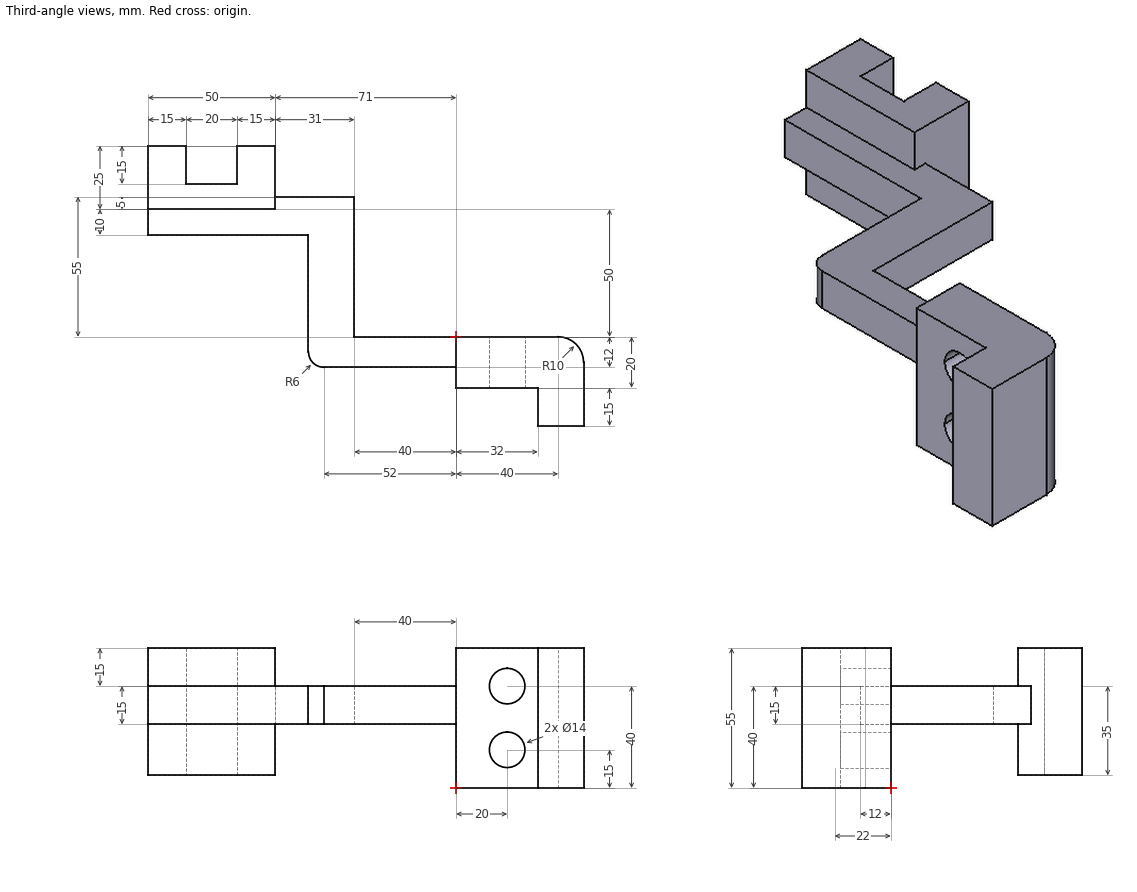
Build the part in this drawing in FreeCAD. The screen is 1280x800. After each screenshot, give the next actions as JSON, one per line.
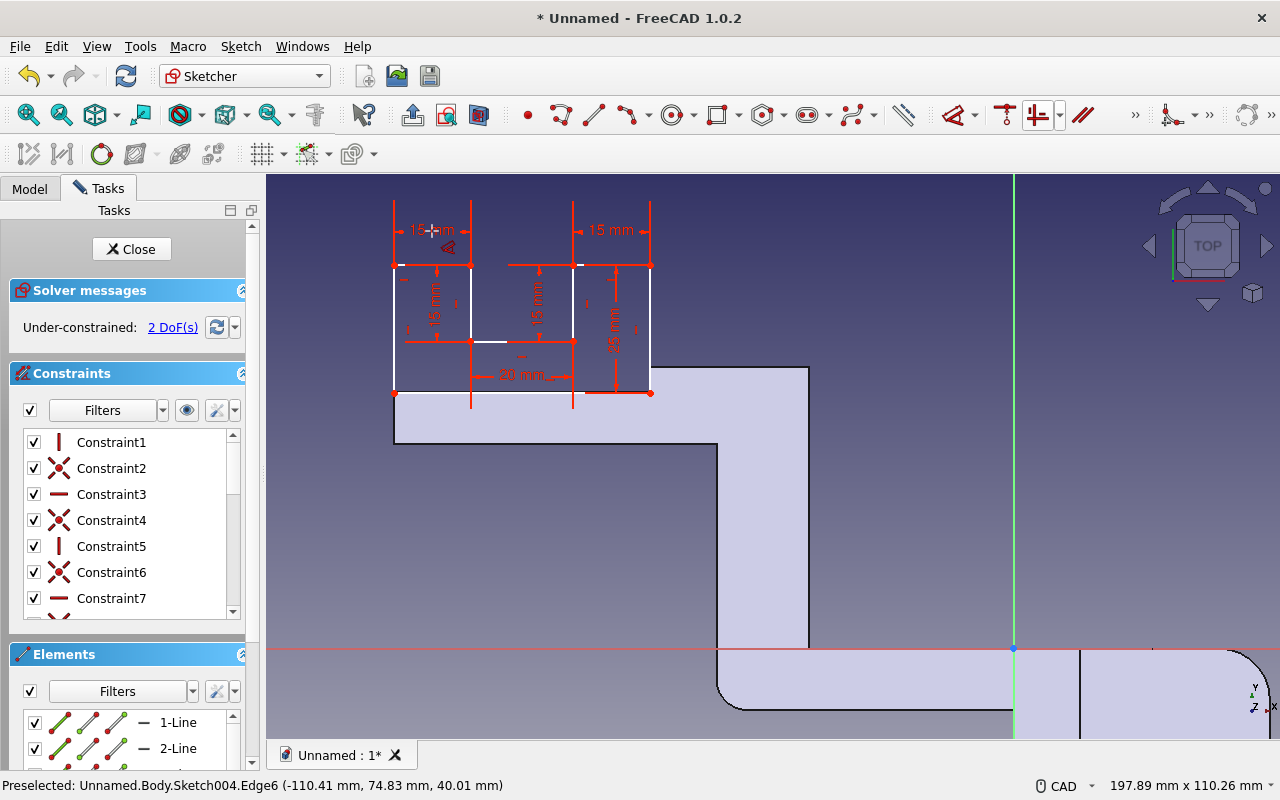
{"action": "left_click", "coordinate": [650, 393]}
{"action": "left_click", "coordinate": [832, 683]}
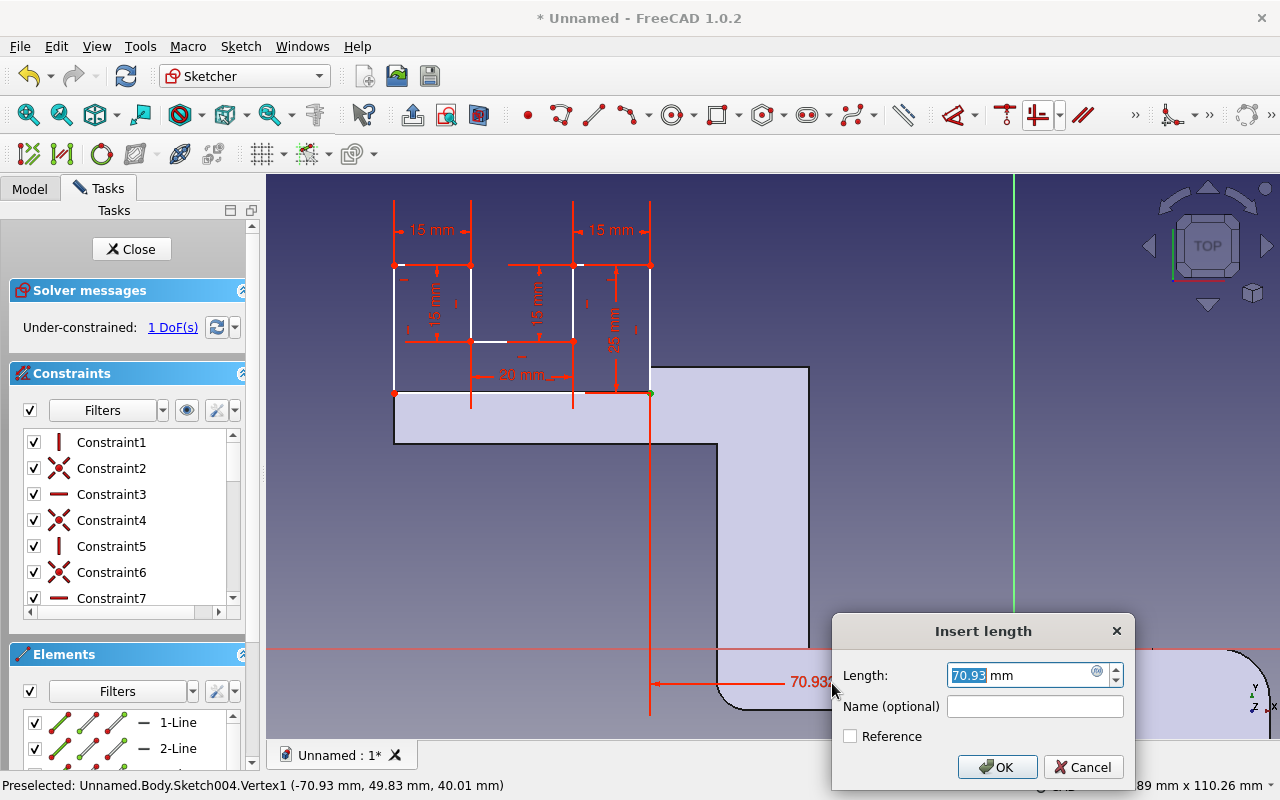
{"action": "type", "text": "71"}
{"action": "key", "text": "Return"}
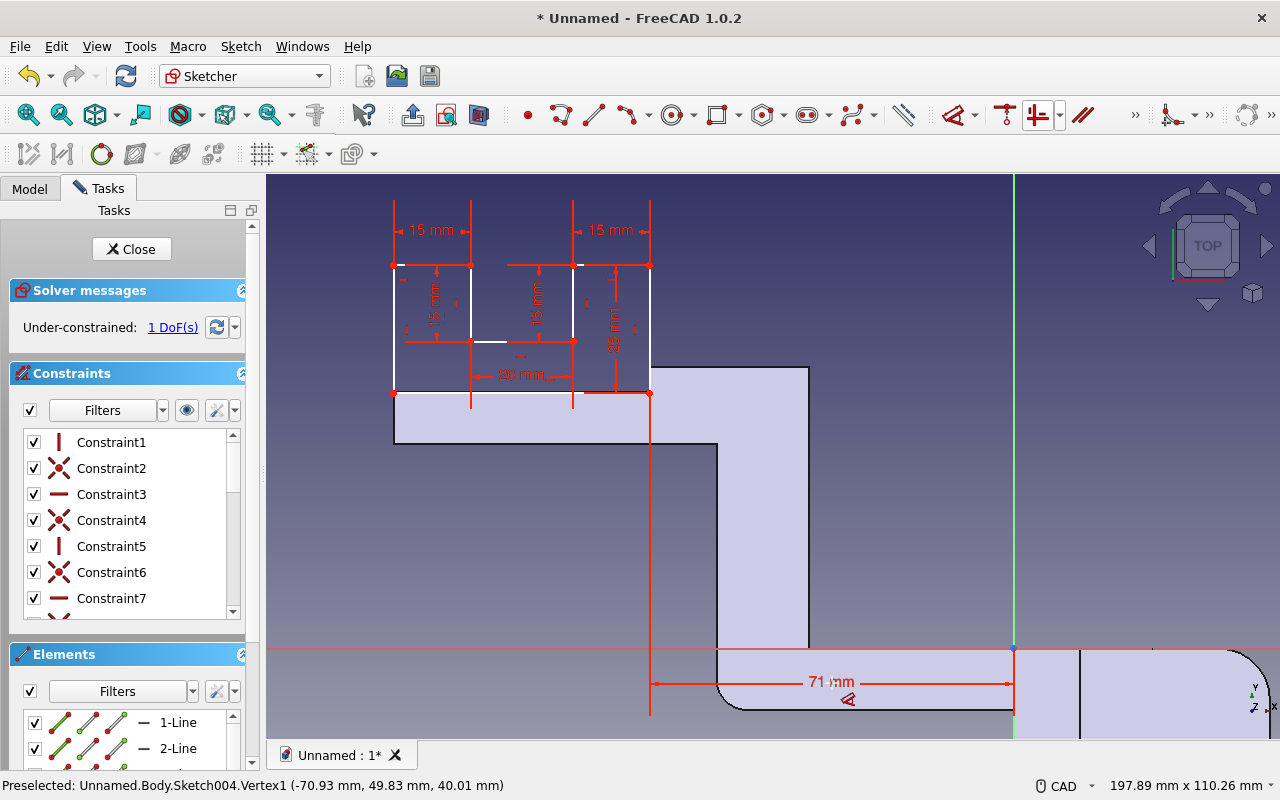
{"action": "left_click", "coordinate": [650, 393]}
{"action": "left_click", "coordinate": [1048, 521]}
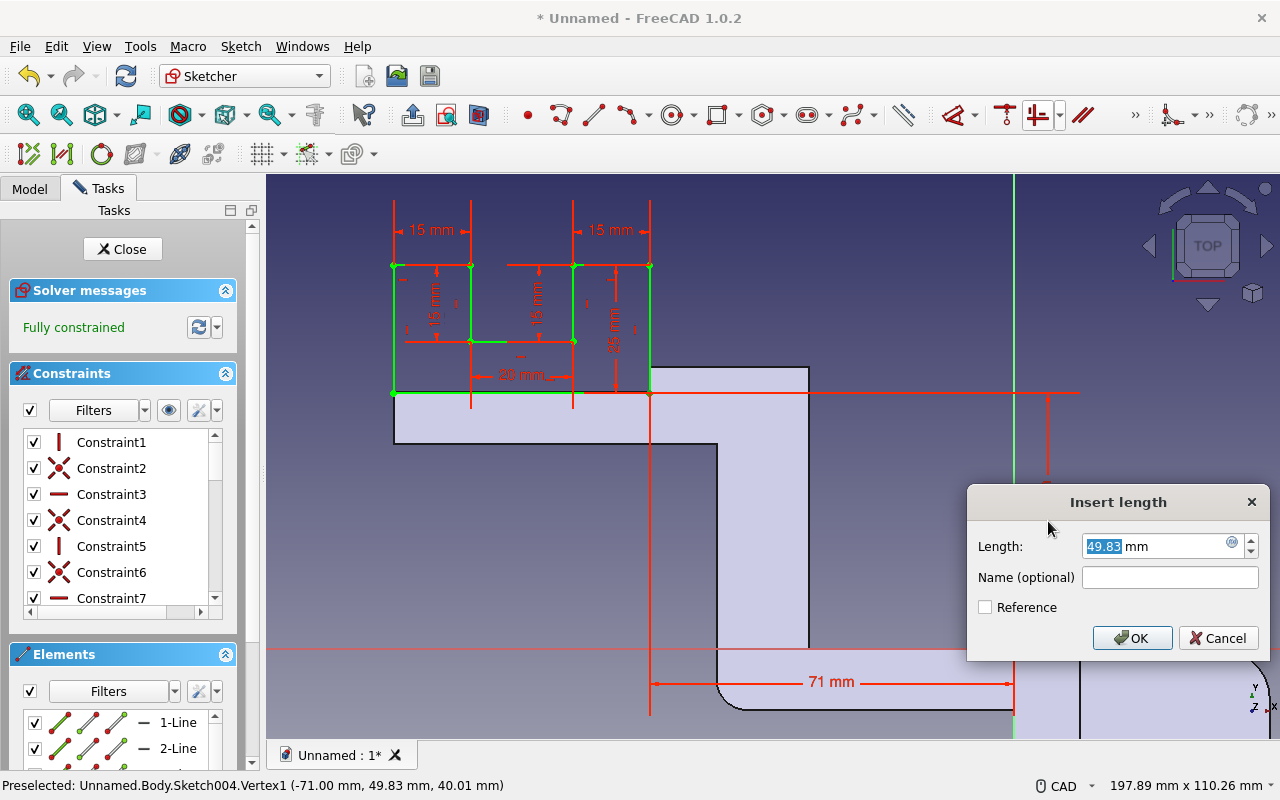
{"action": "type", "text": "50"}
{"action": "key", "text": "Return"}
{"action": "key", "text": "Escape"}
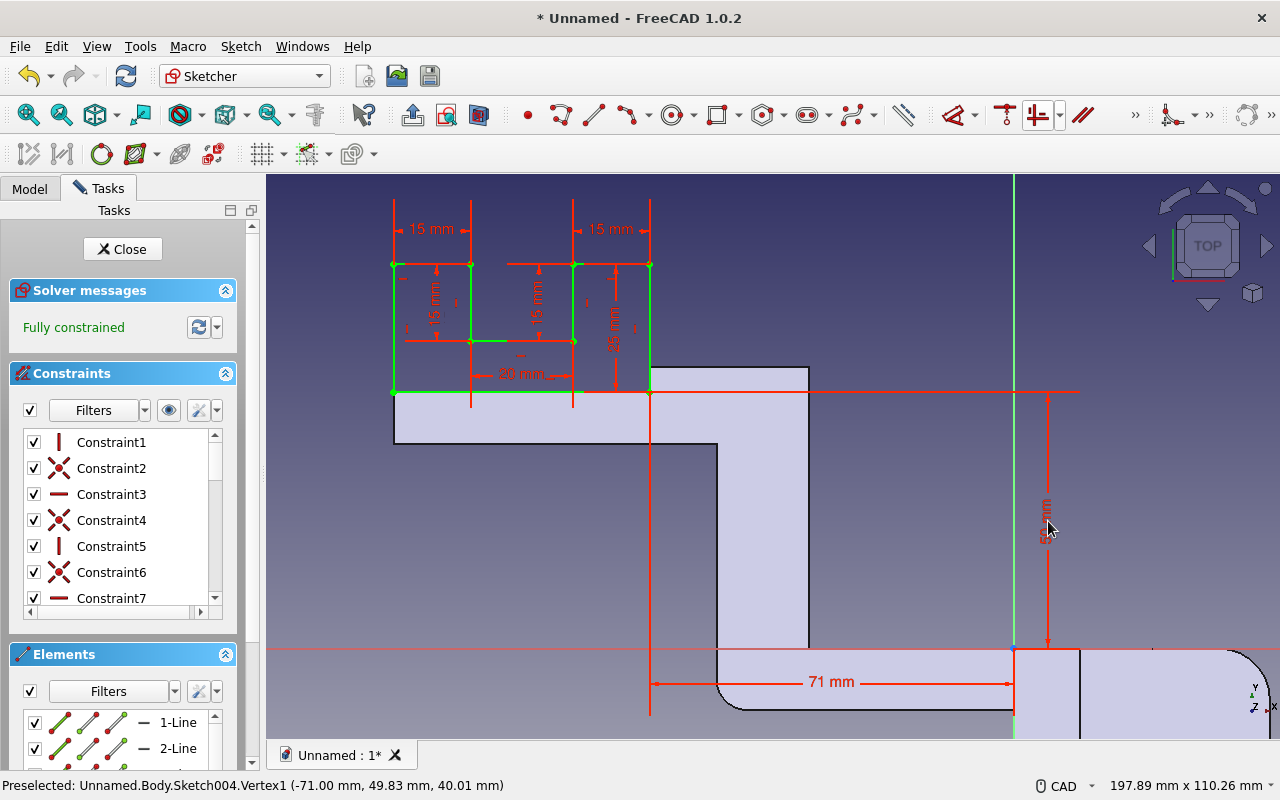
{"action": "left_click", "coordinate": [123, 249]}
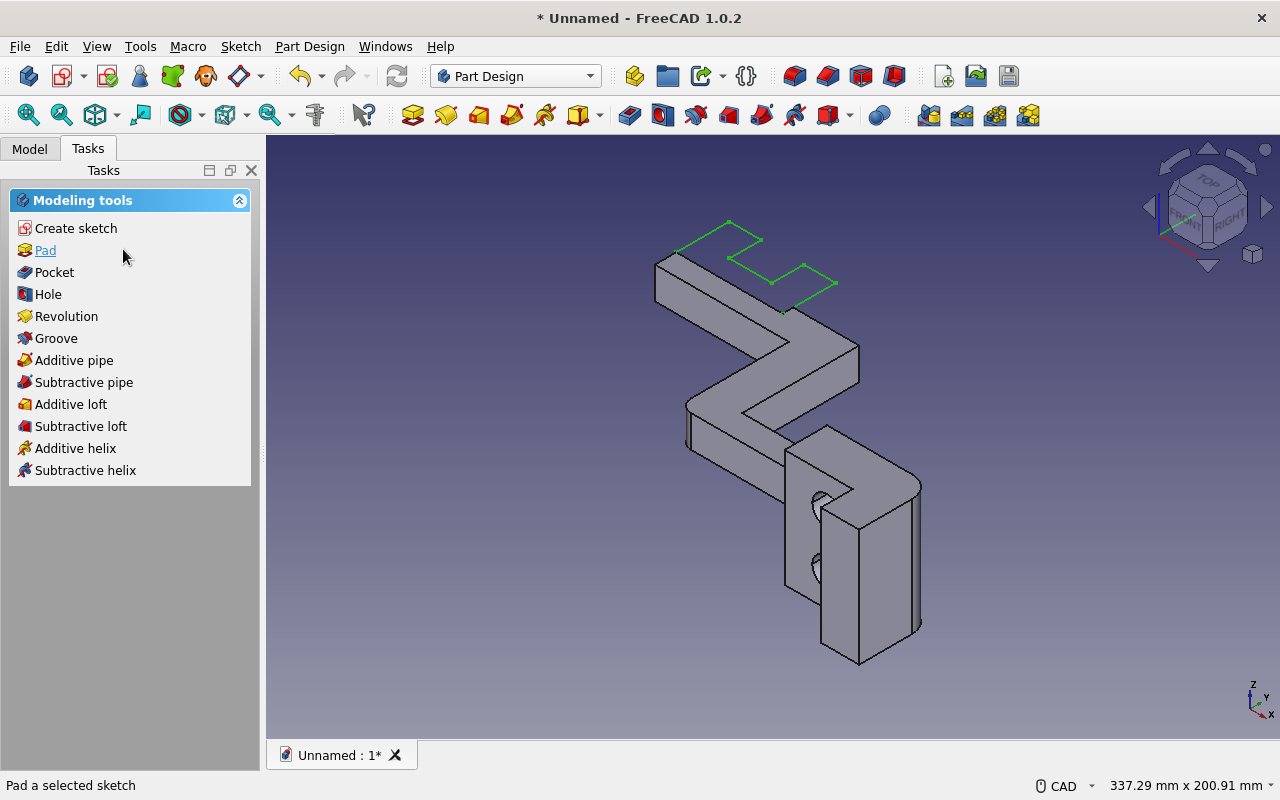
{"action": "left_click", "coordinate": [413, 116]}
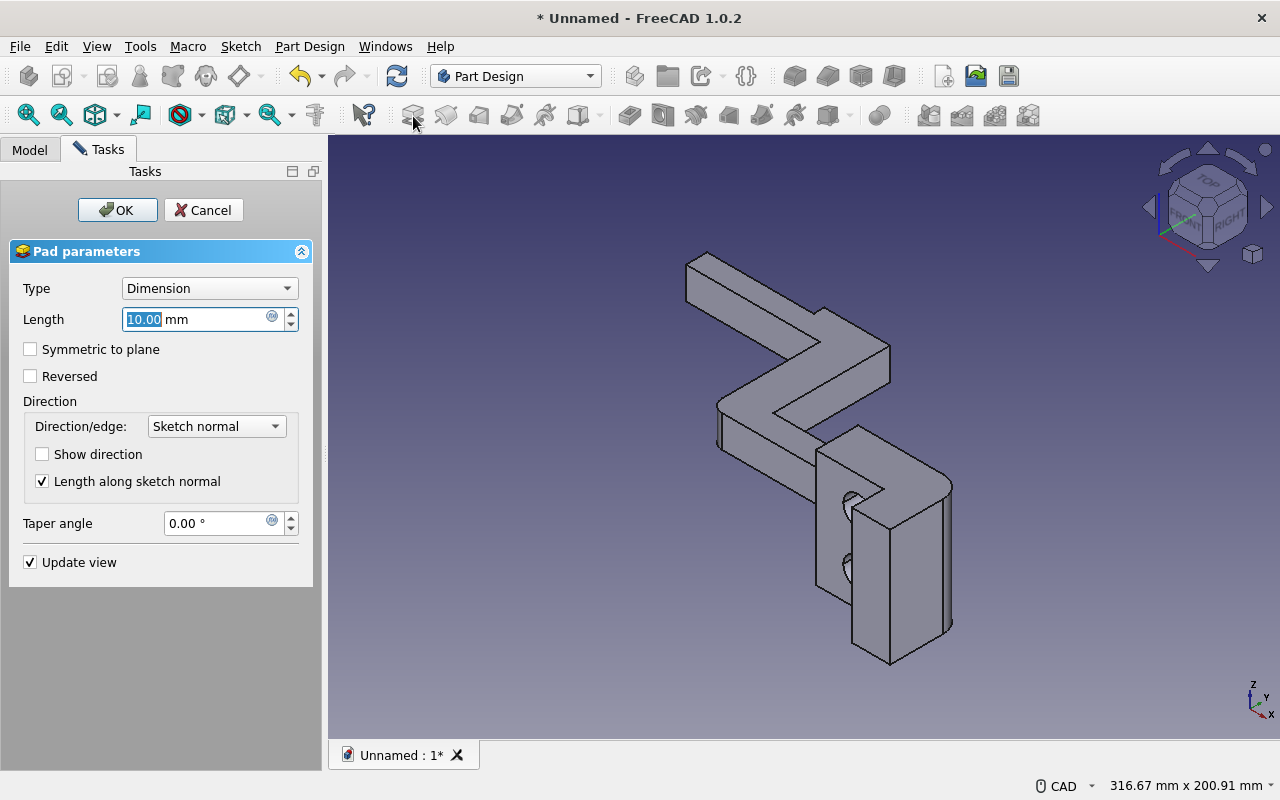
{"action": "type", "text": "35"}
{"action": "key", "text": "Tab"}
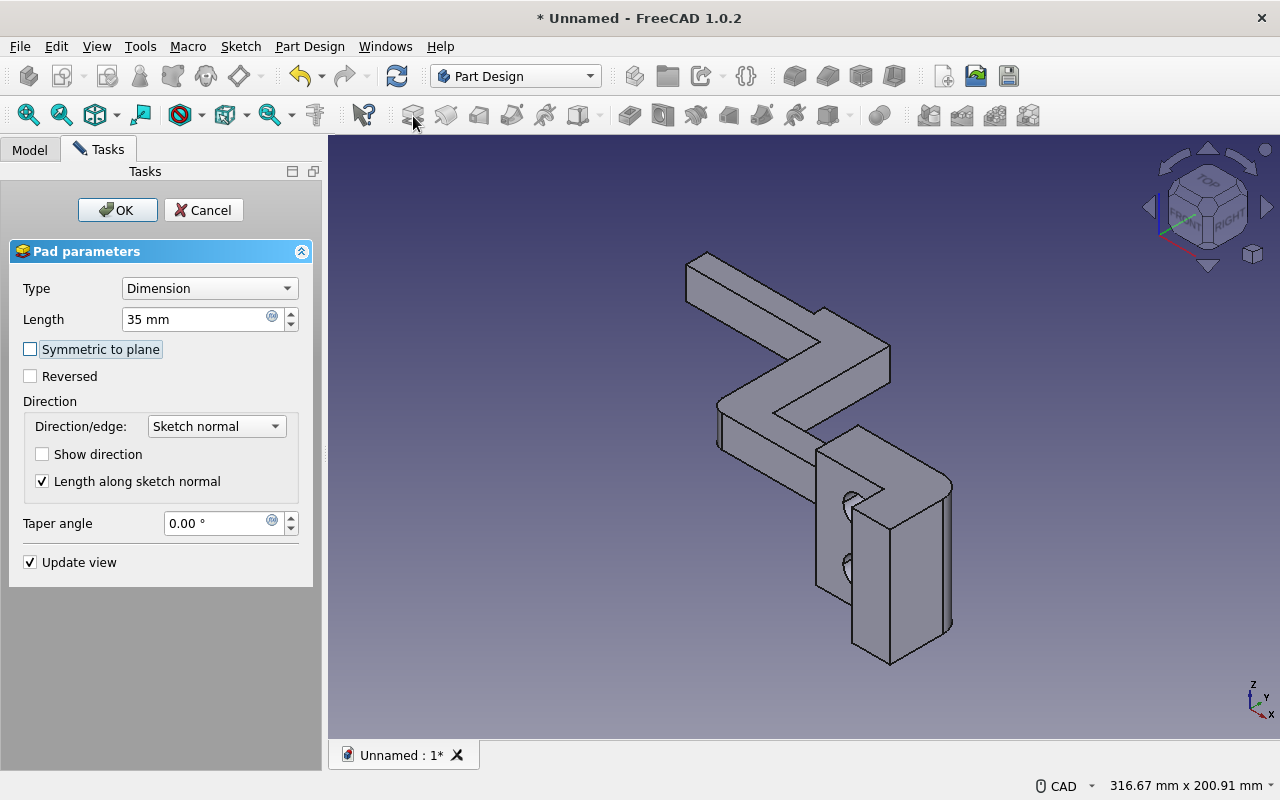
{"action": "left_click", "coordinate": [31, 376]}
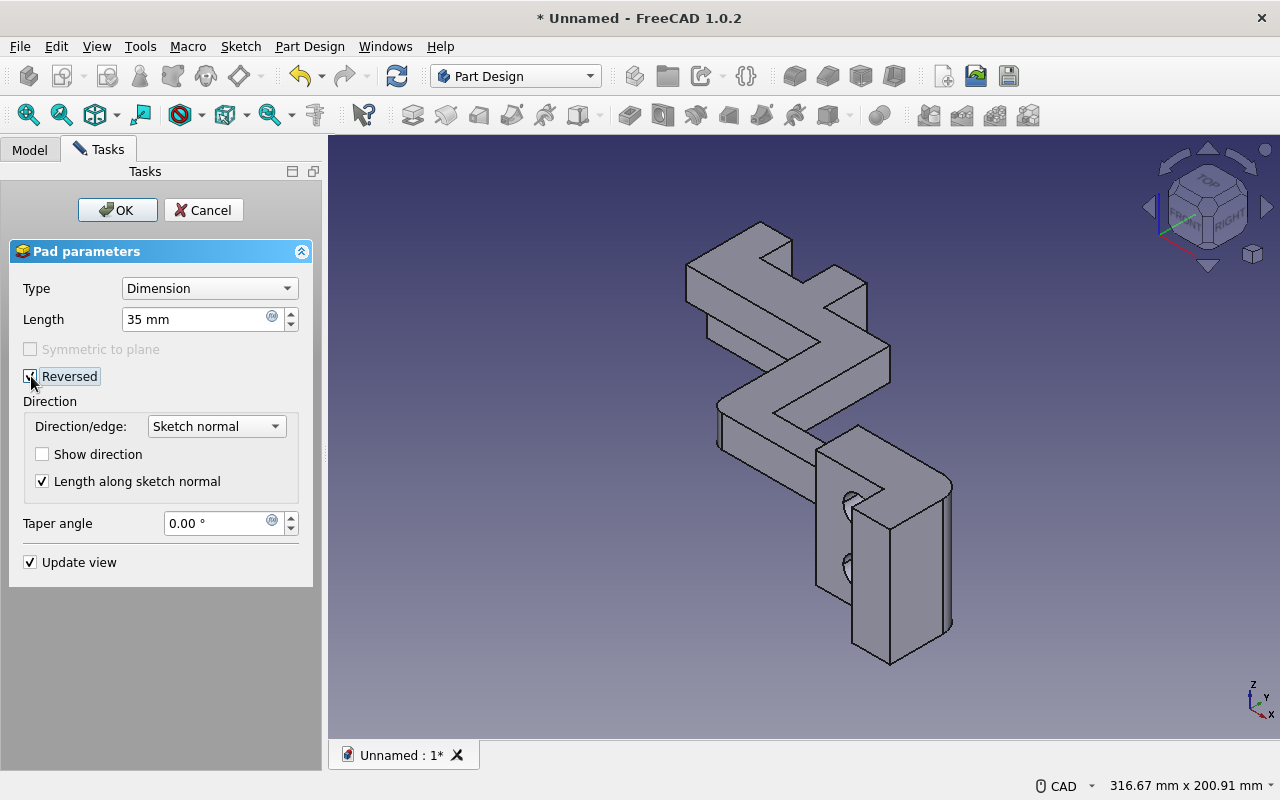
{"action": "left_click", "coordinate": [118, 210]}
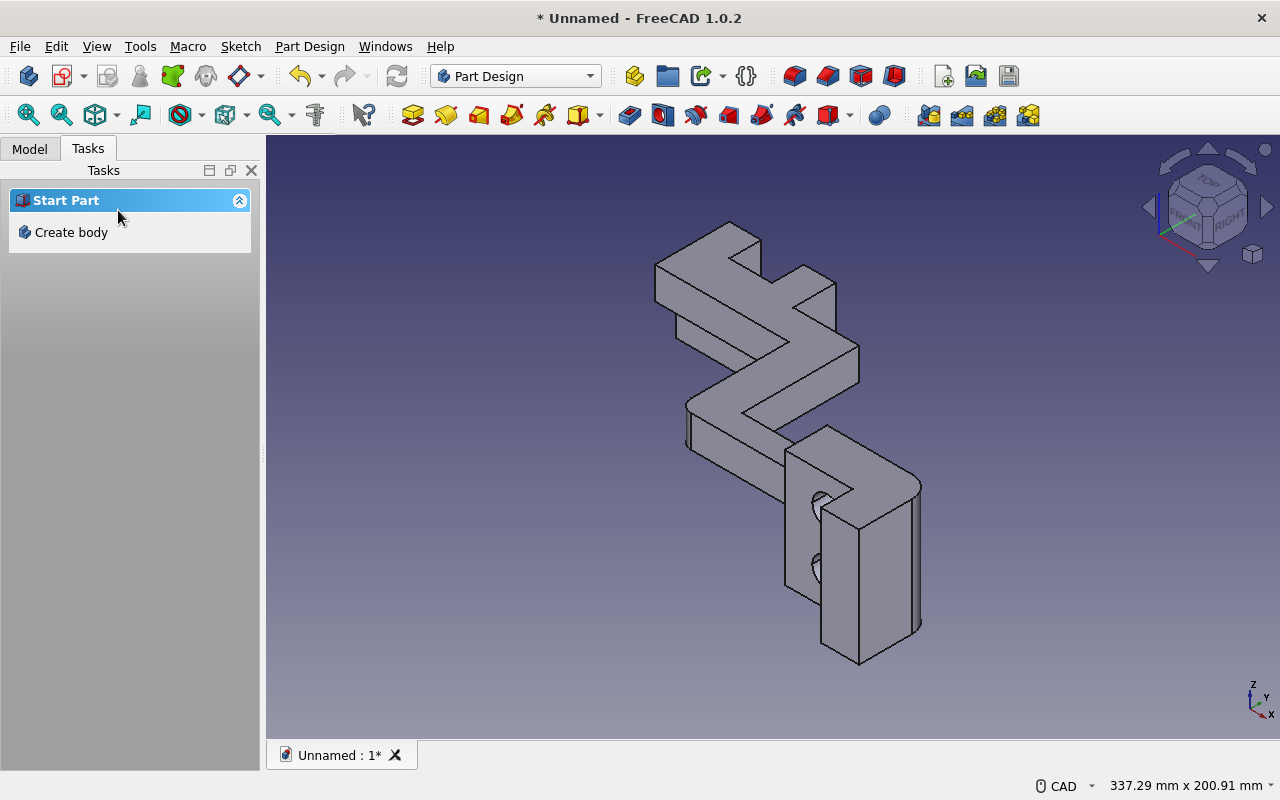
{"action": "left_click", "coordinate": [708, 254]}